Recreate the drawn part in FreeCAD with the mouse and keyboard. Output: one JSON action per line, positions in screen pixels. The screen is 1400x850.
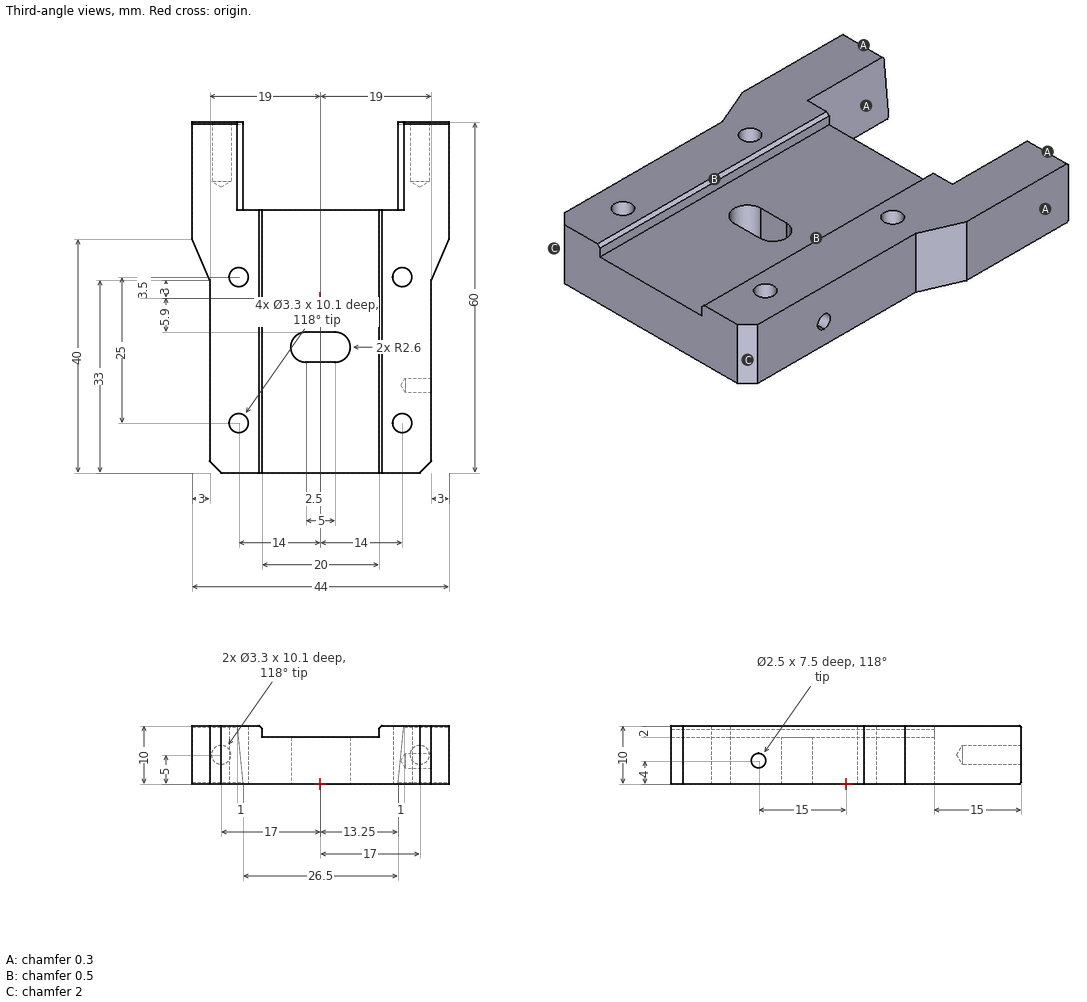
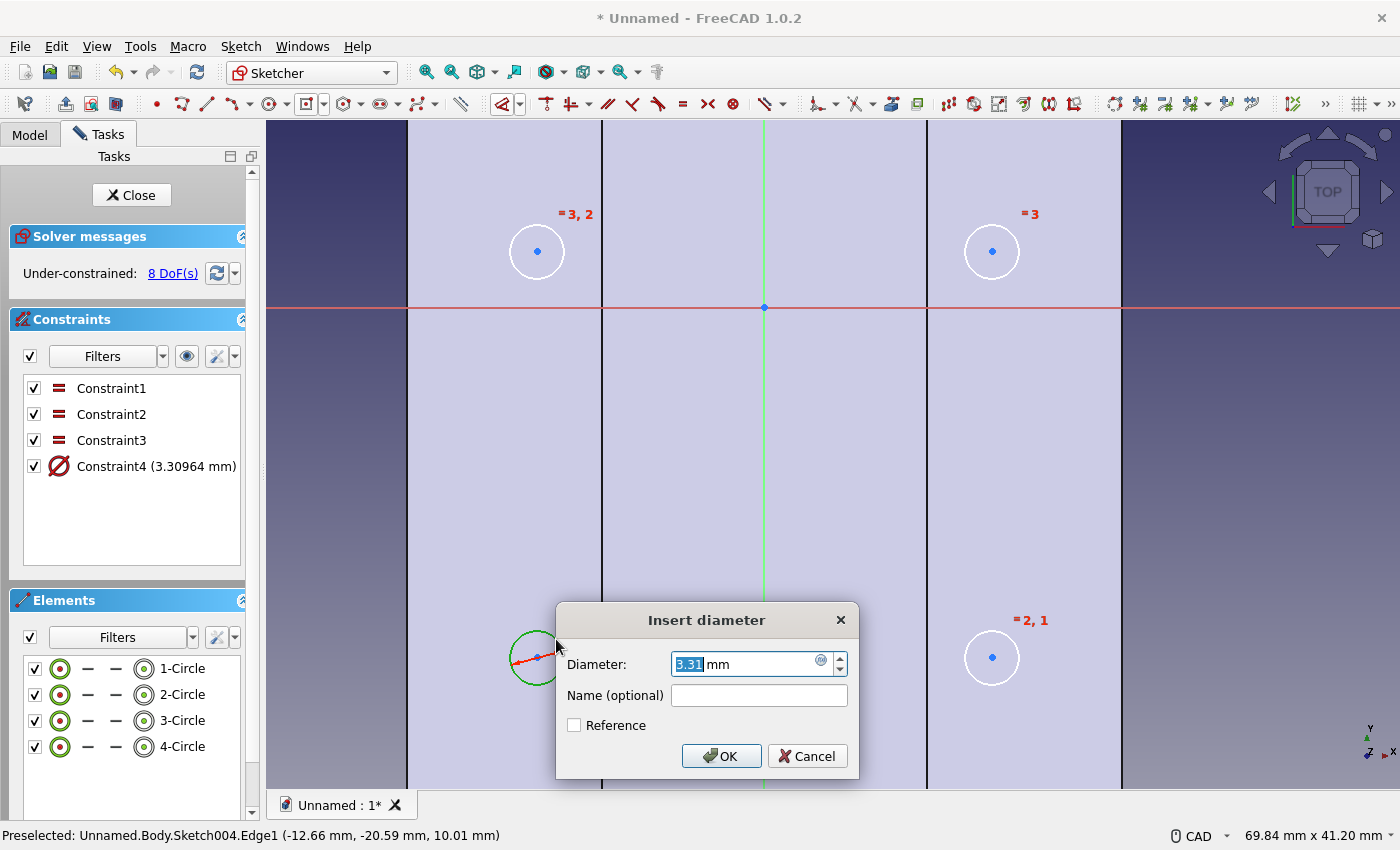
{"action": "type", "text": "3.3"}
{"action": "key", "text": "Return"}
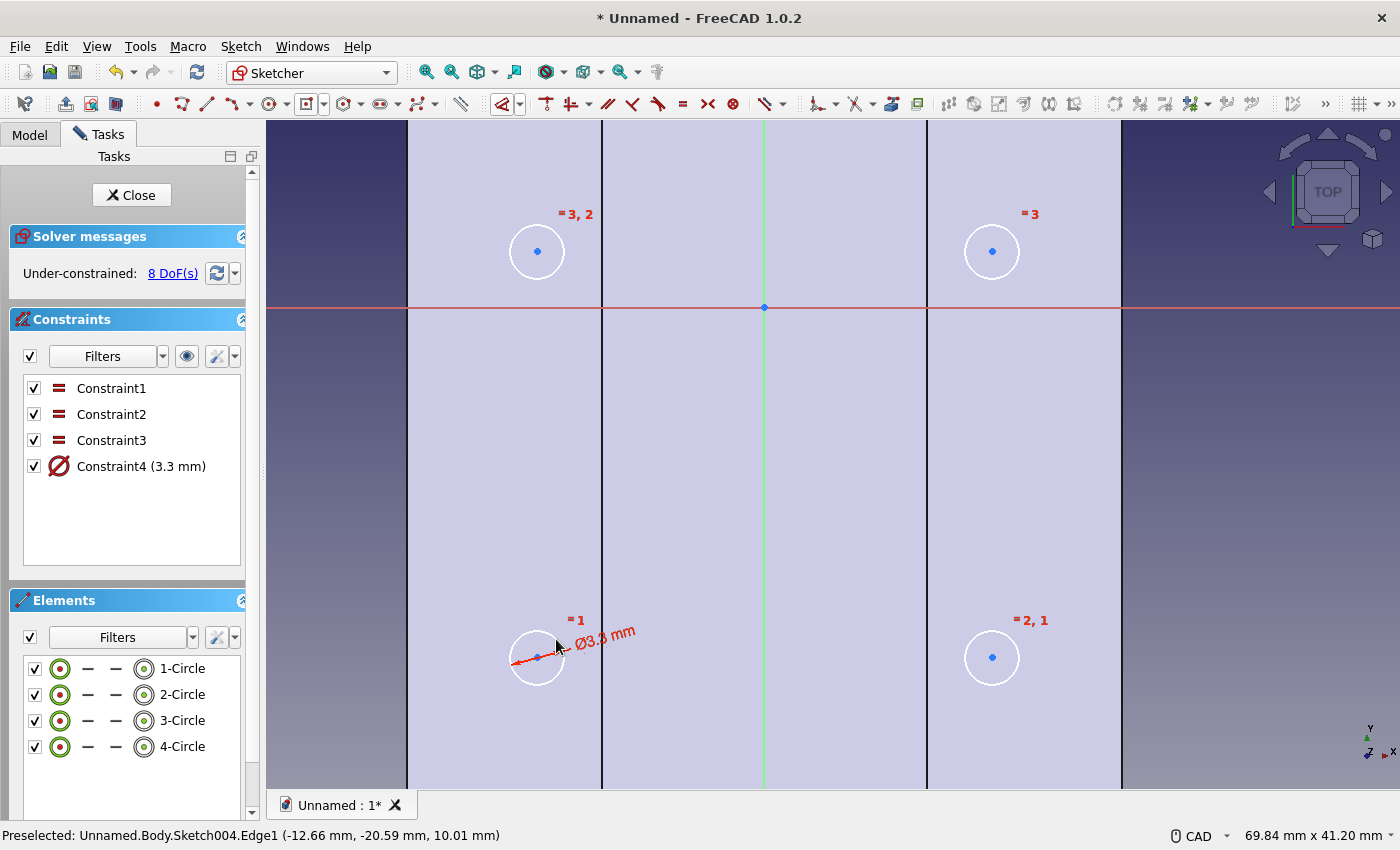
{"action": "left_click", "coordinate": [537, 658]}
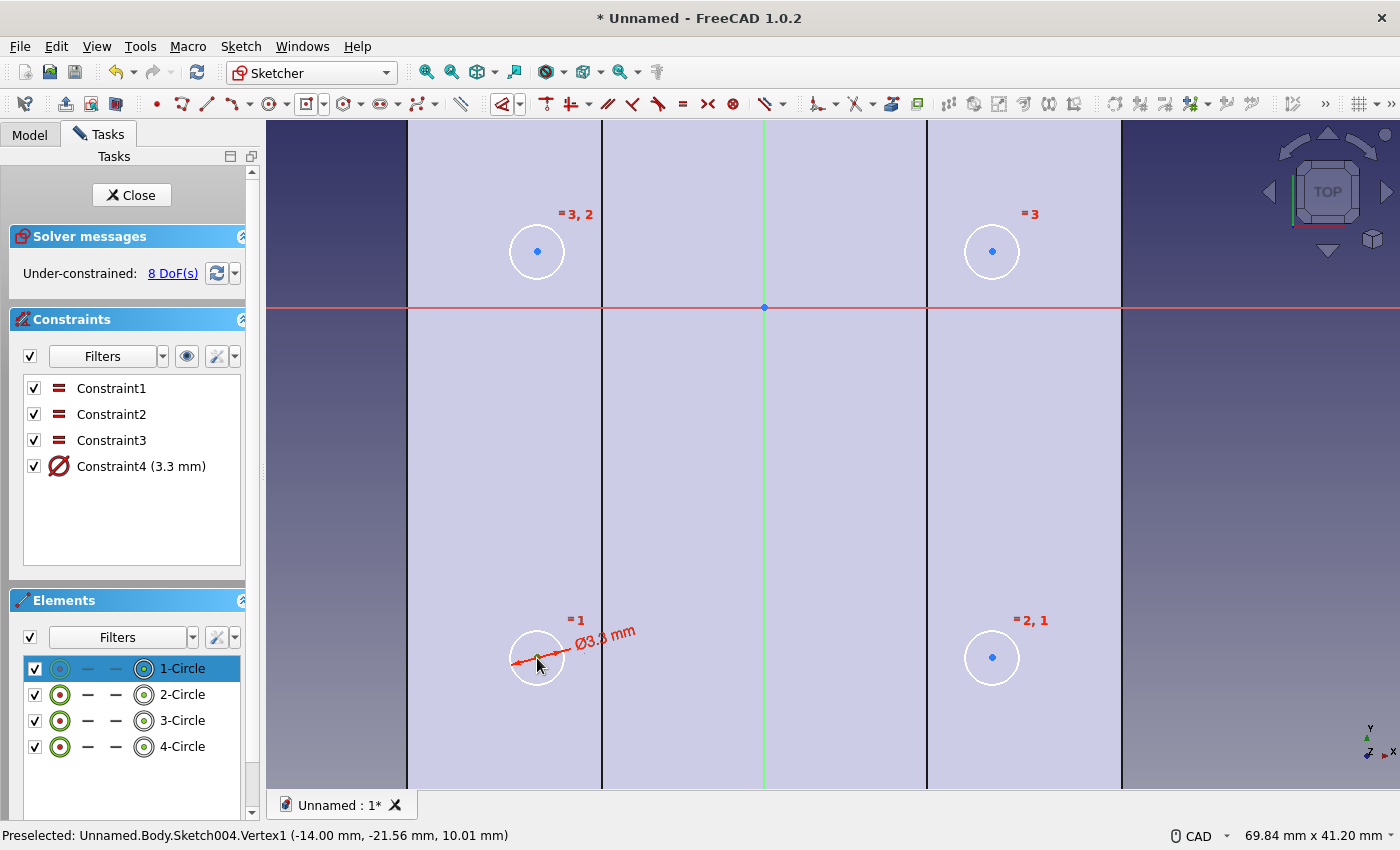
{"action": "key", "text": "l"}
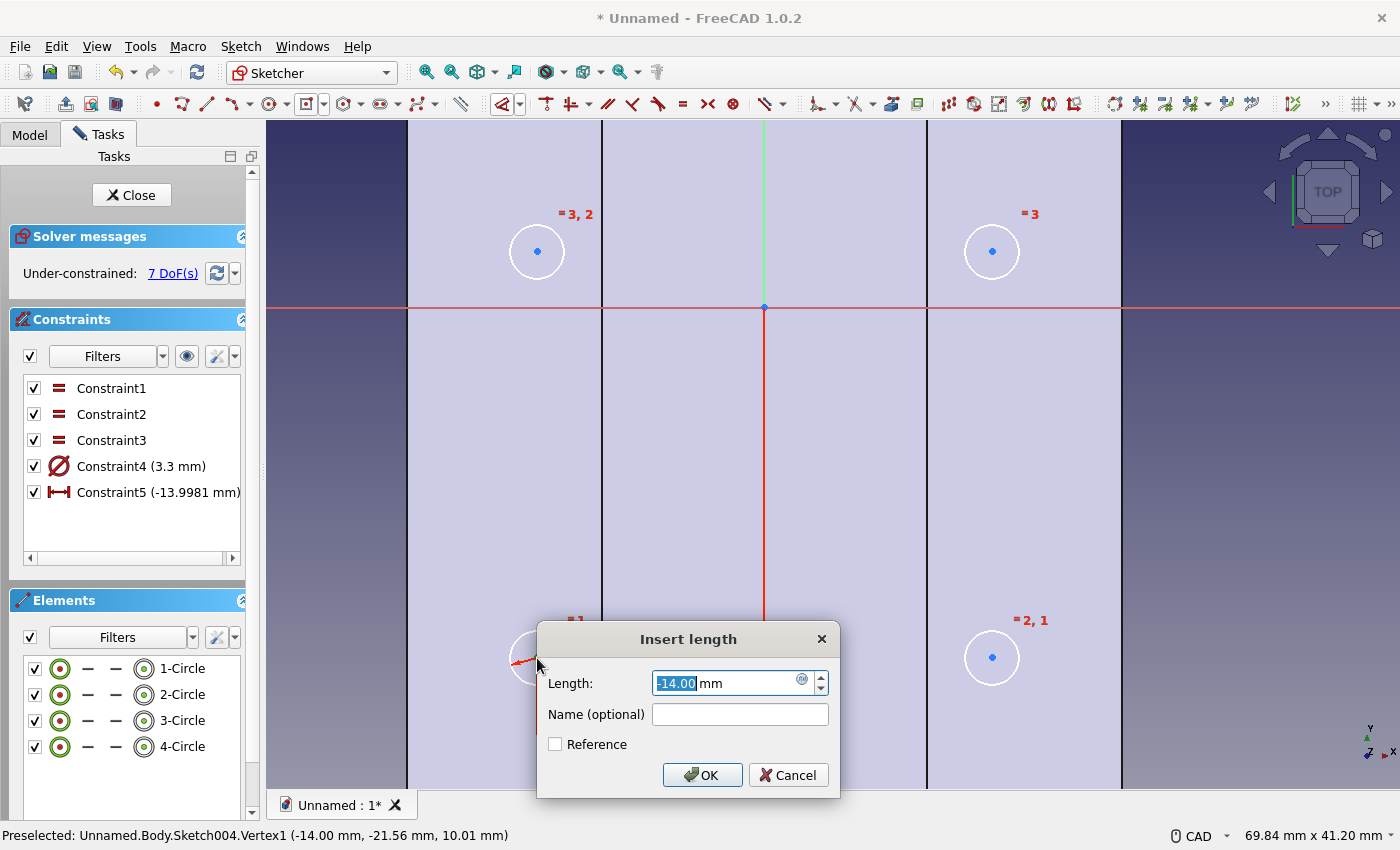
{"action": "type", "text": "-14"}
{"action": "key", "text": "Return"}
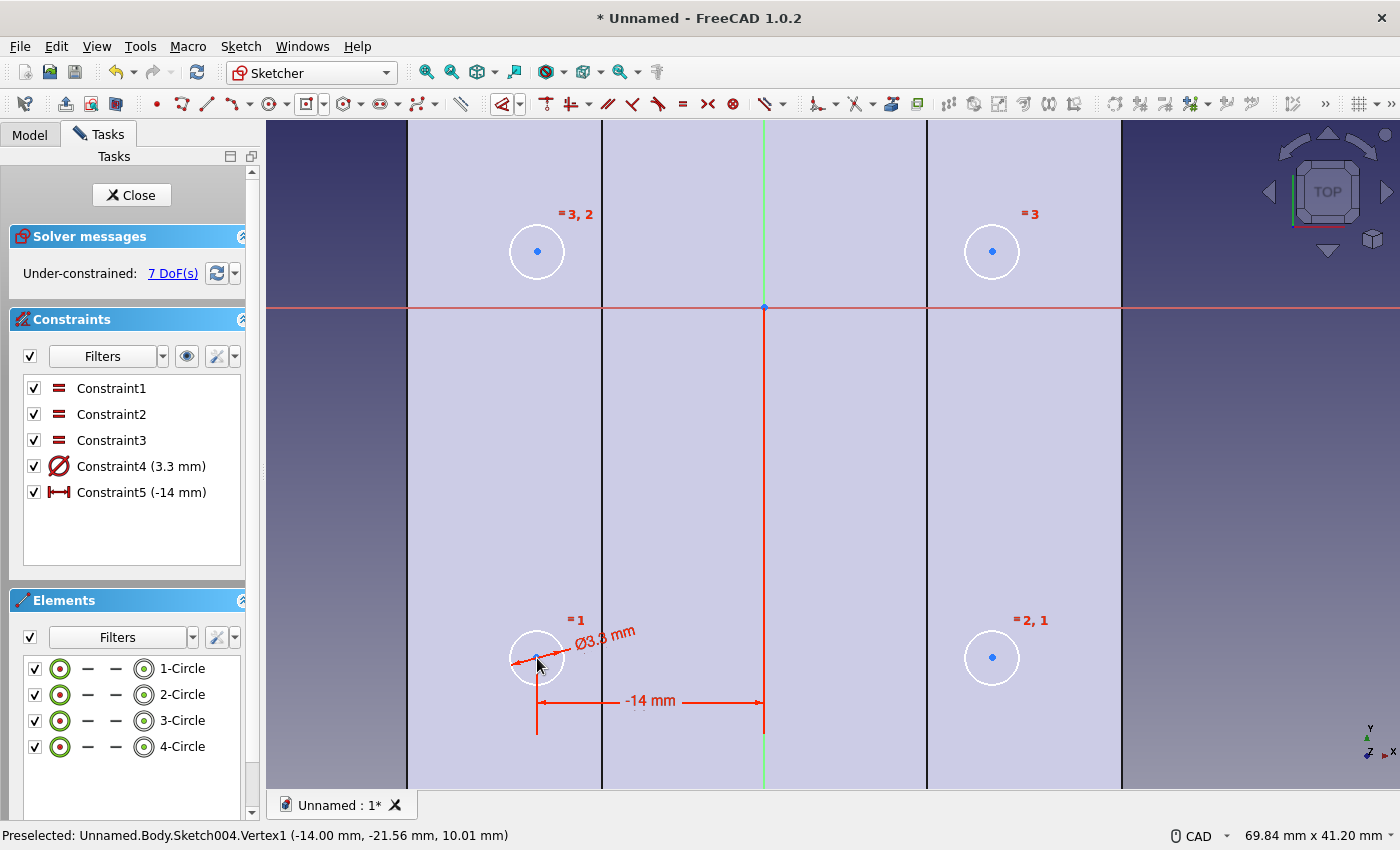
{"action": "left_click", "coordinate": [992, 658]}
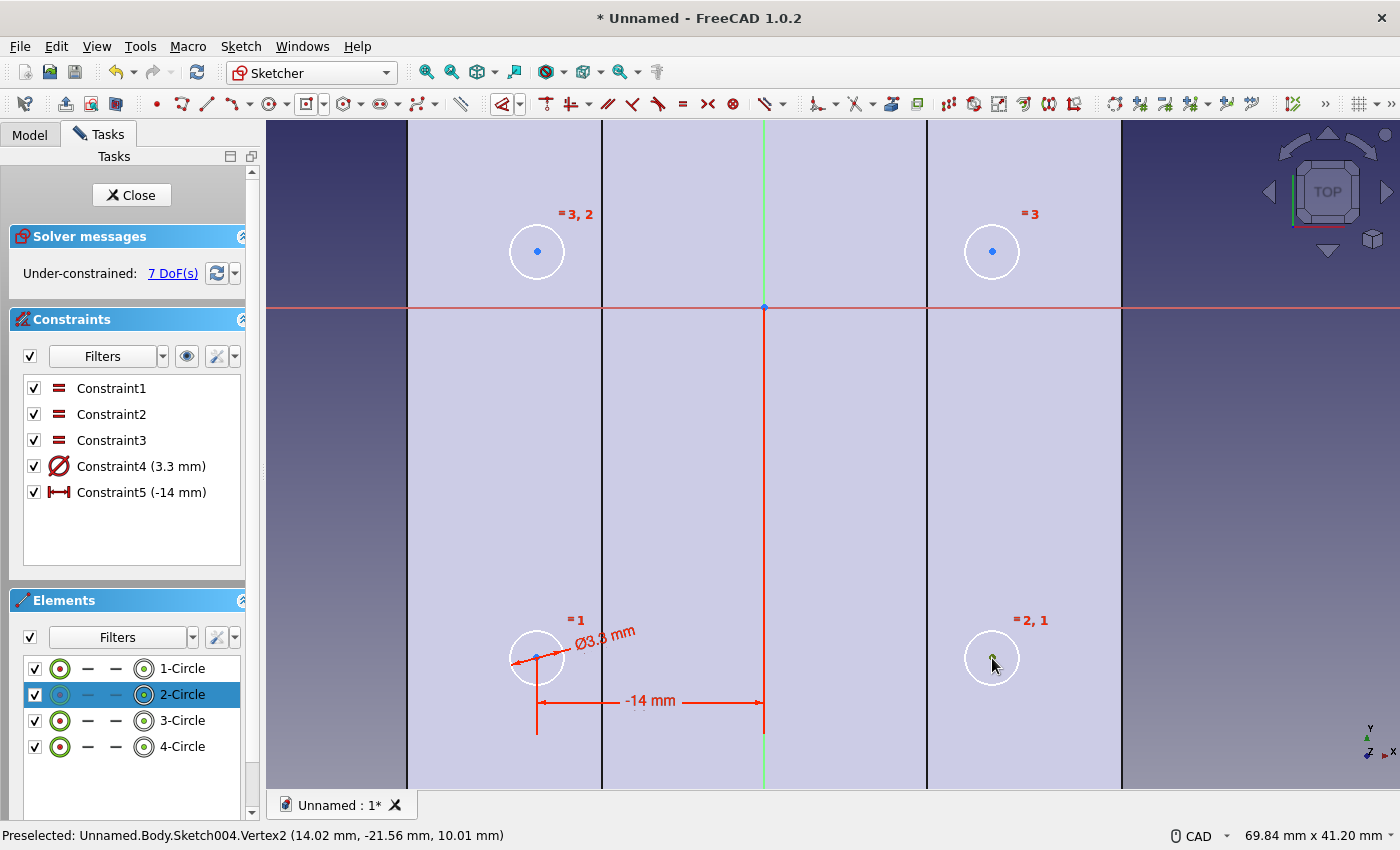
{"action": "key", "text": "l"}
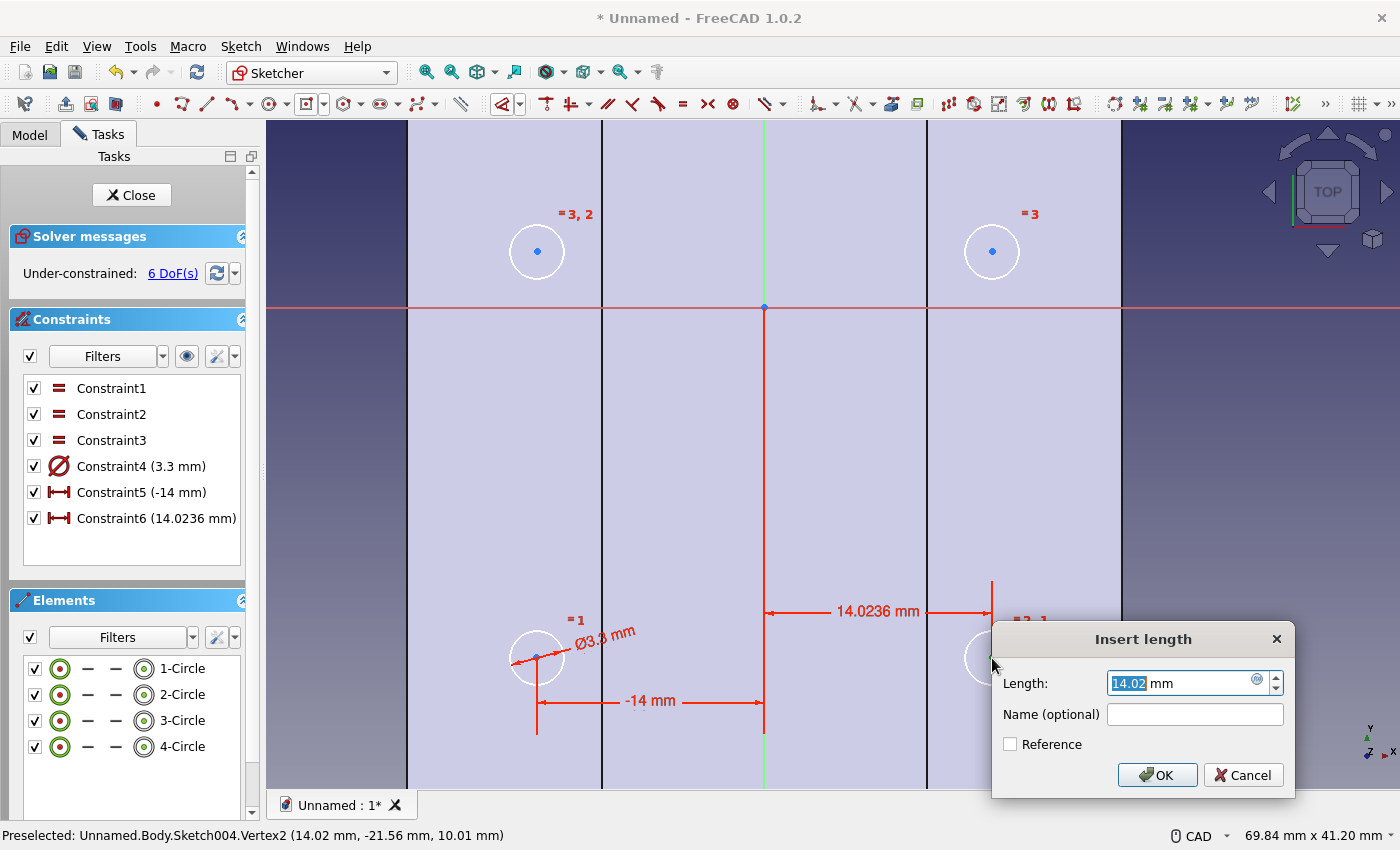
{"action": "type", "text": "14"}
{"action": "key", "text": "Return"}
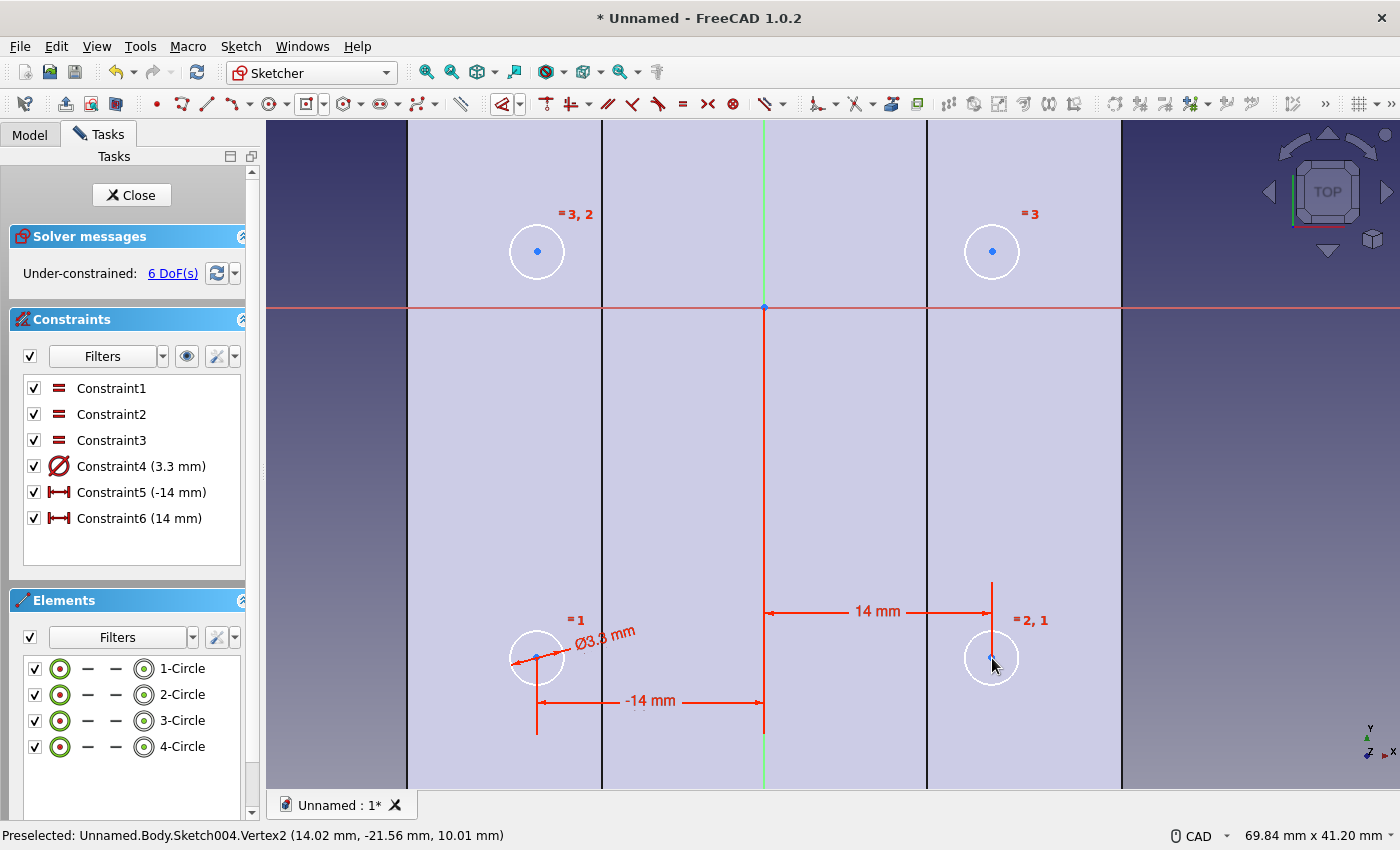
{"action": "left_click", "coordinate": [537, 252]}